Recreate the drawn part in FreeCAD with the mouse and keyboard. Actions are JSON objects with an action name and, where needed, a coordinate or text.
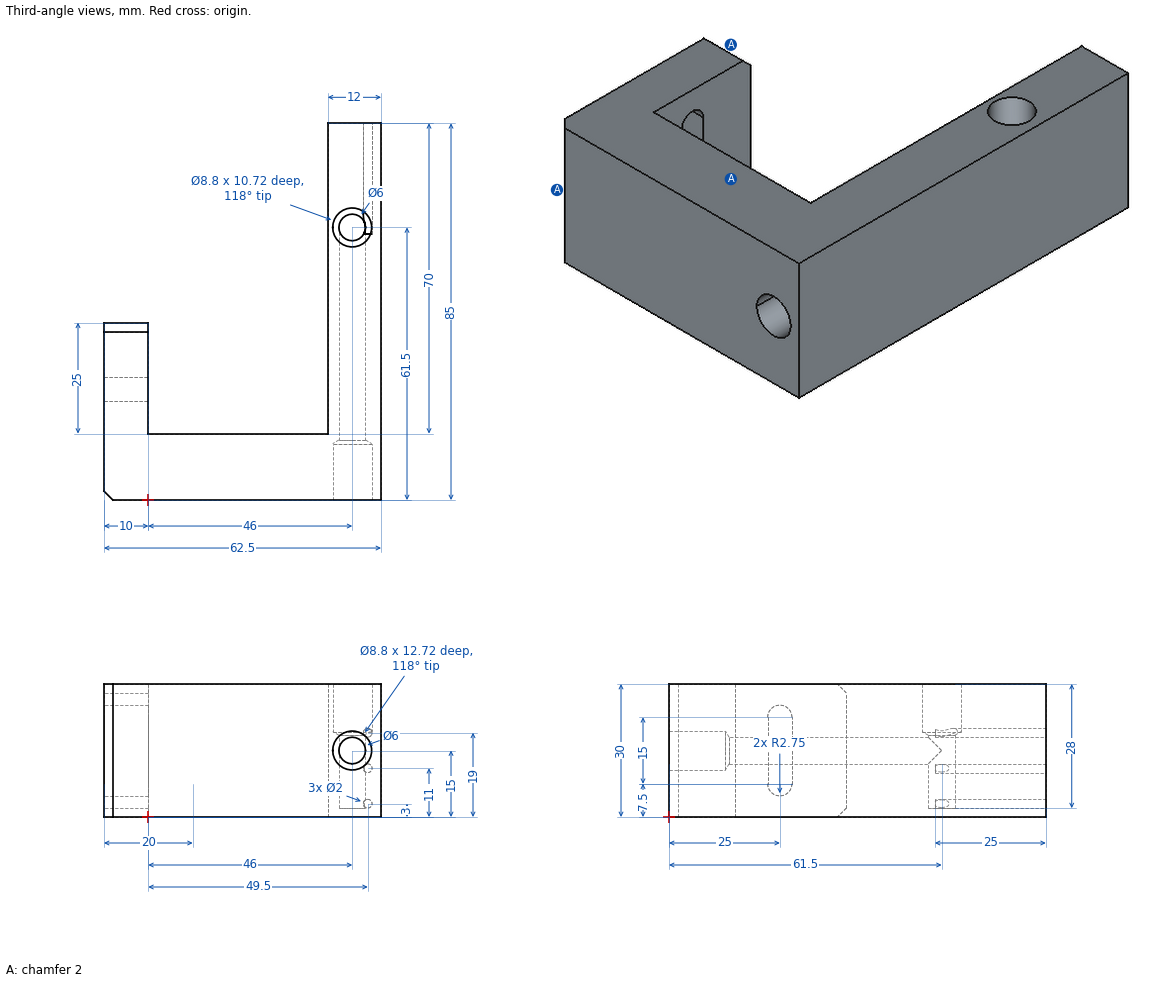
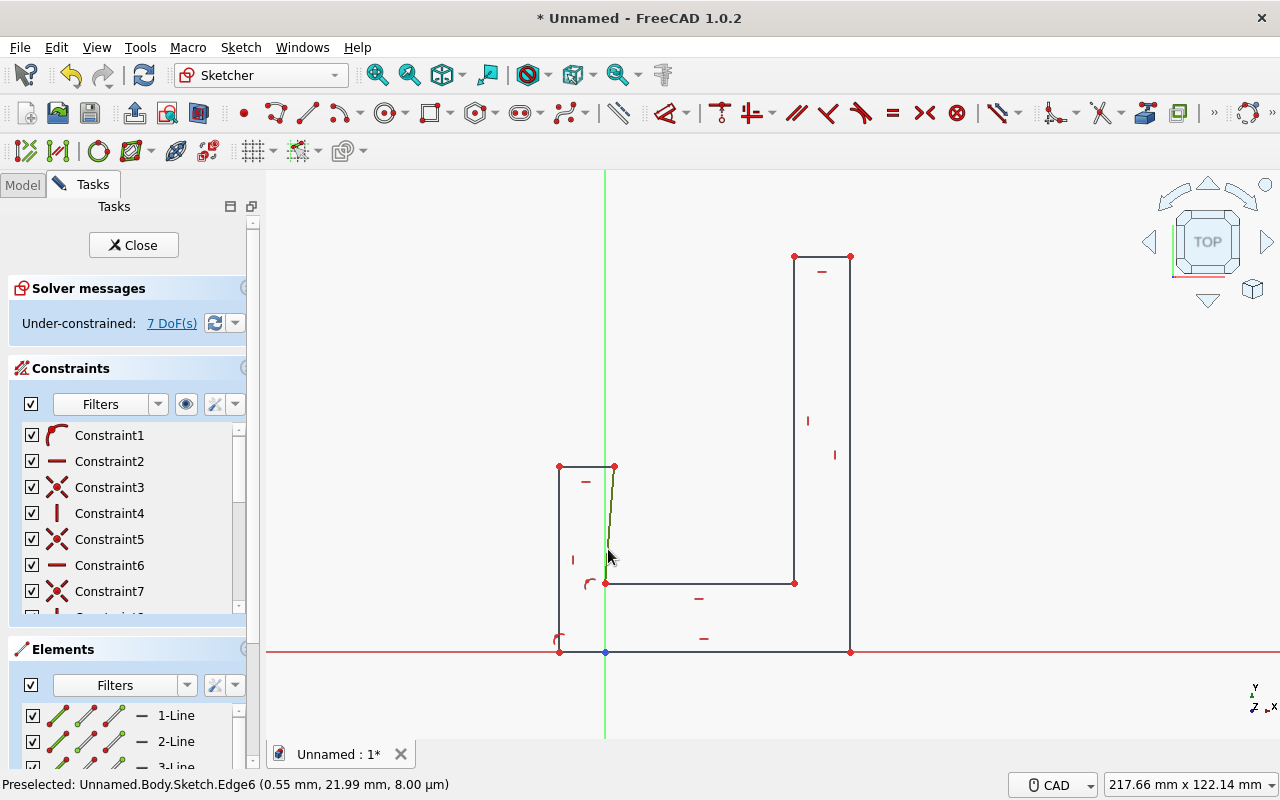
{"action": "left_click", "coordinate": [774, 114]}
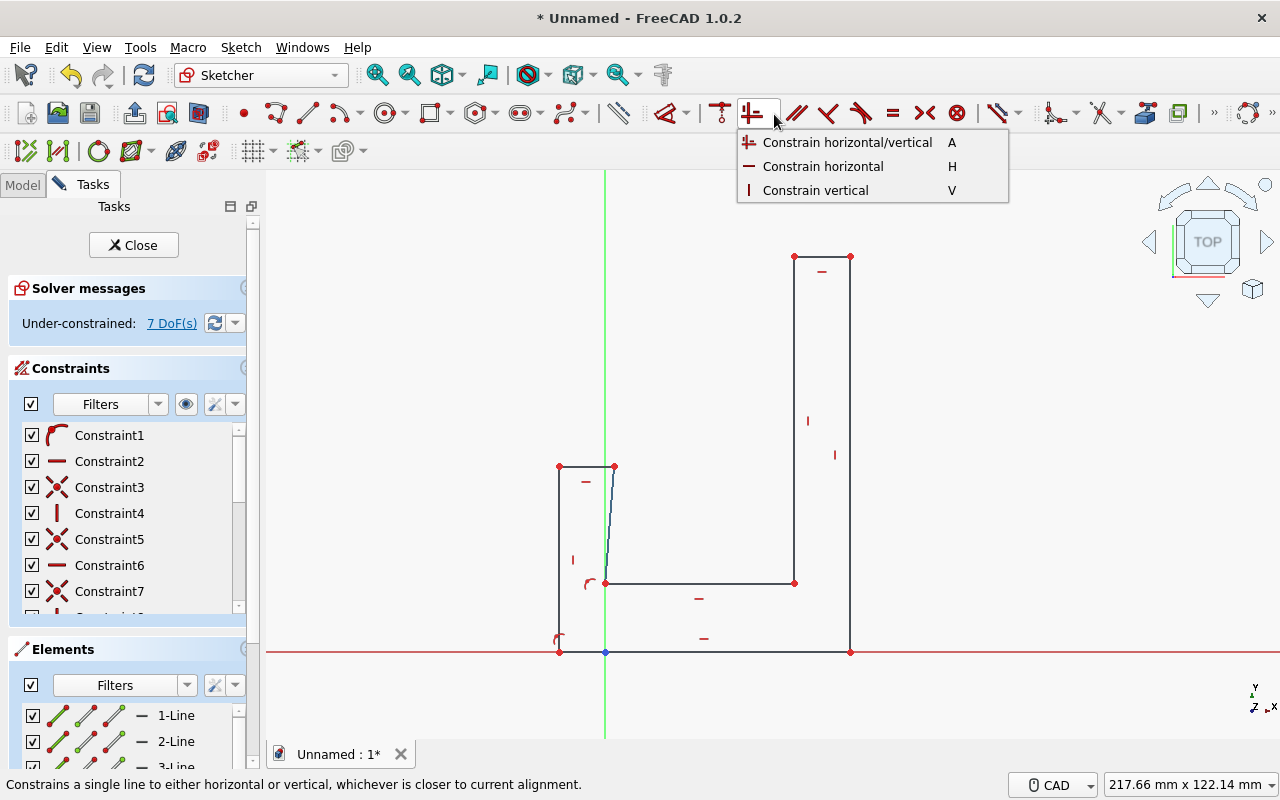
{"action": "left_click", "coordinate": [873, 190]}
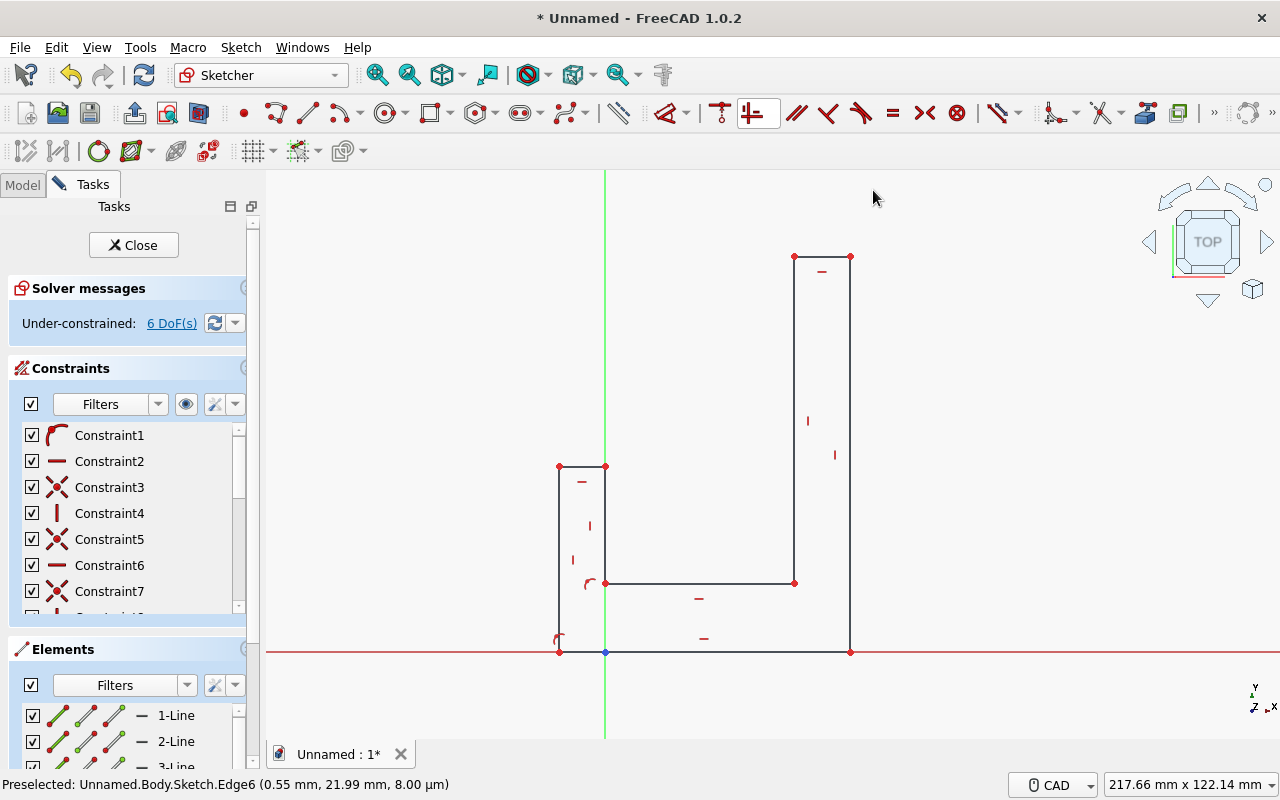
{"action": "left_click", "coordinate": [666, 114]}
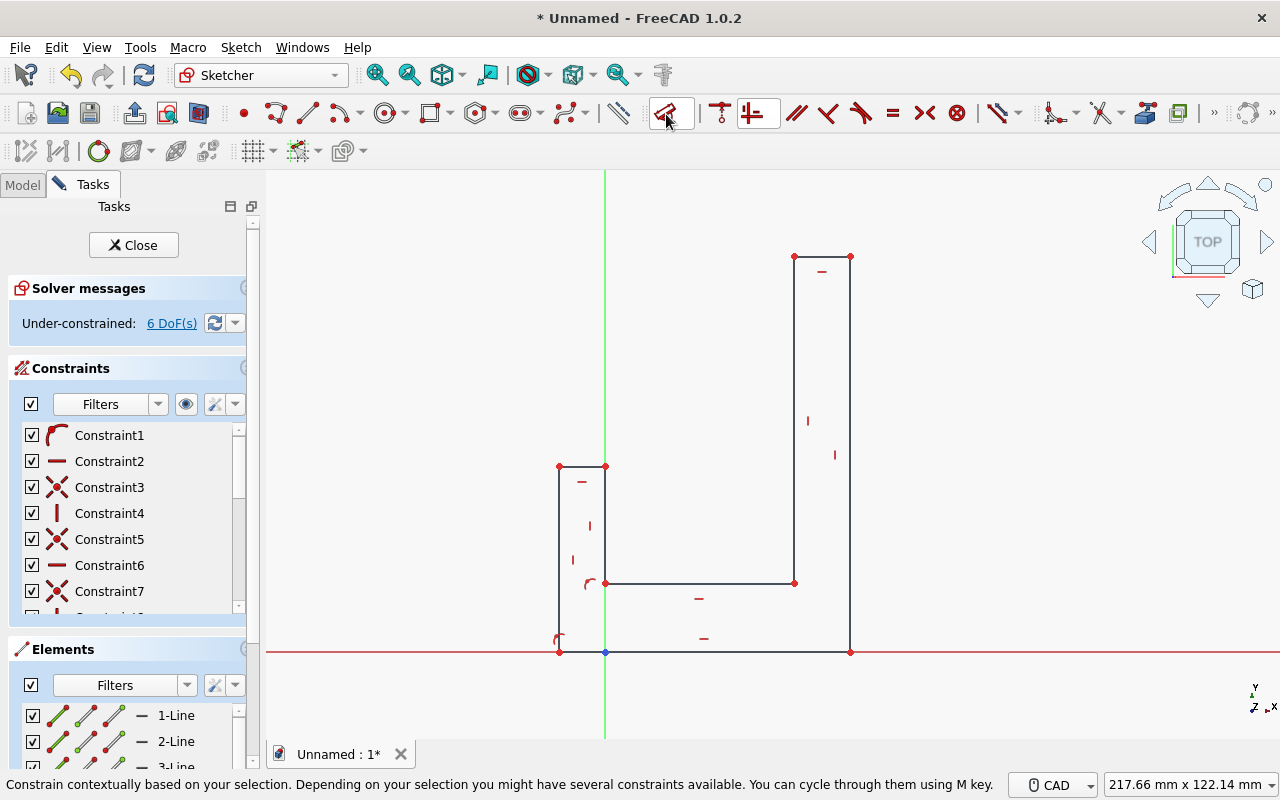
{"action": "left_click", "coordinate": [850, 534]}
{"action": "left_click", "coordinate": [884, 455]}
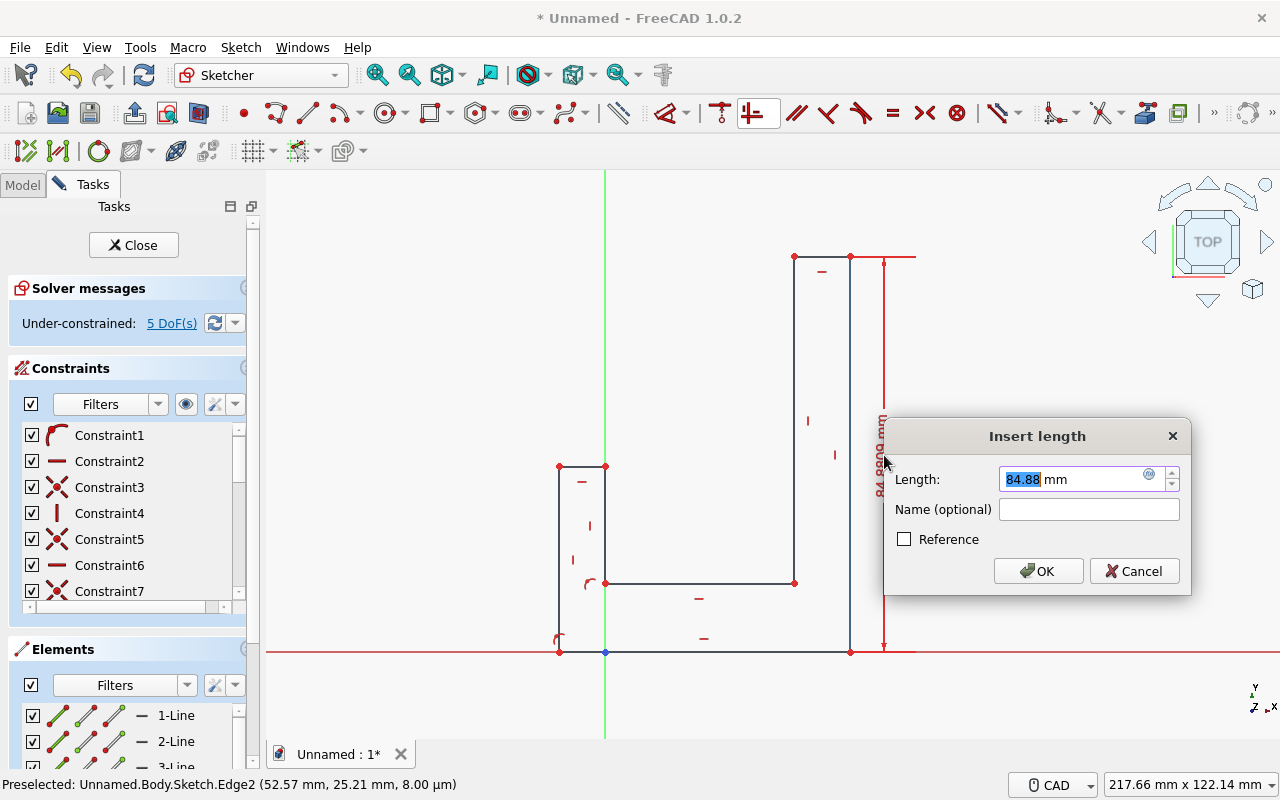
{"action": "type", "text": "85"}
{"action": "key", "text": "Return"}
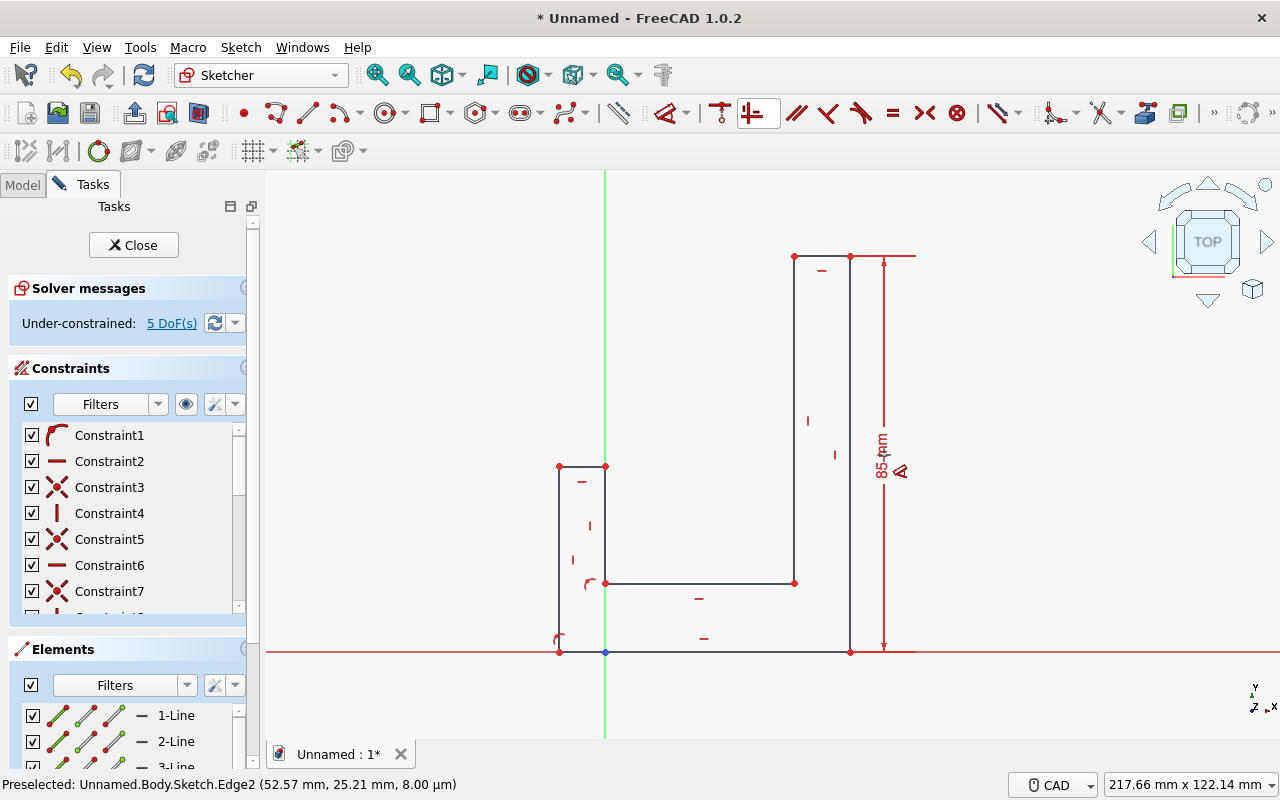
{"action": "left_click", "coordinate": [833, 256]}
{"action": "left_click", "coordinate": [822, 222]}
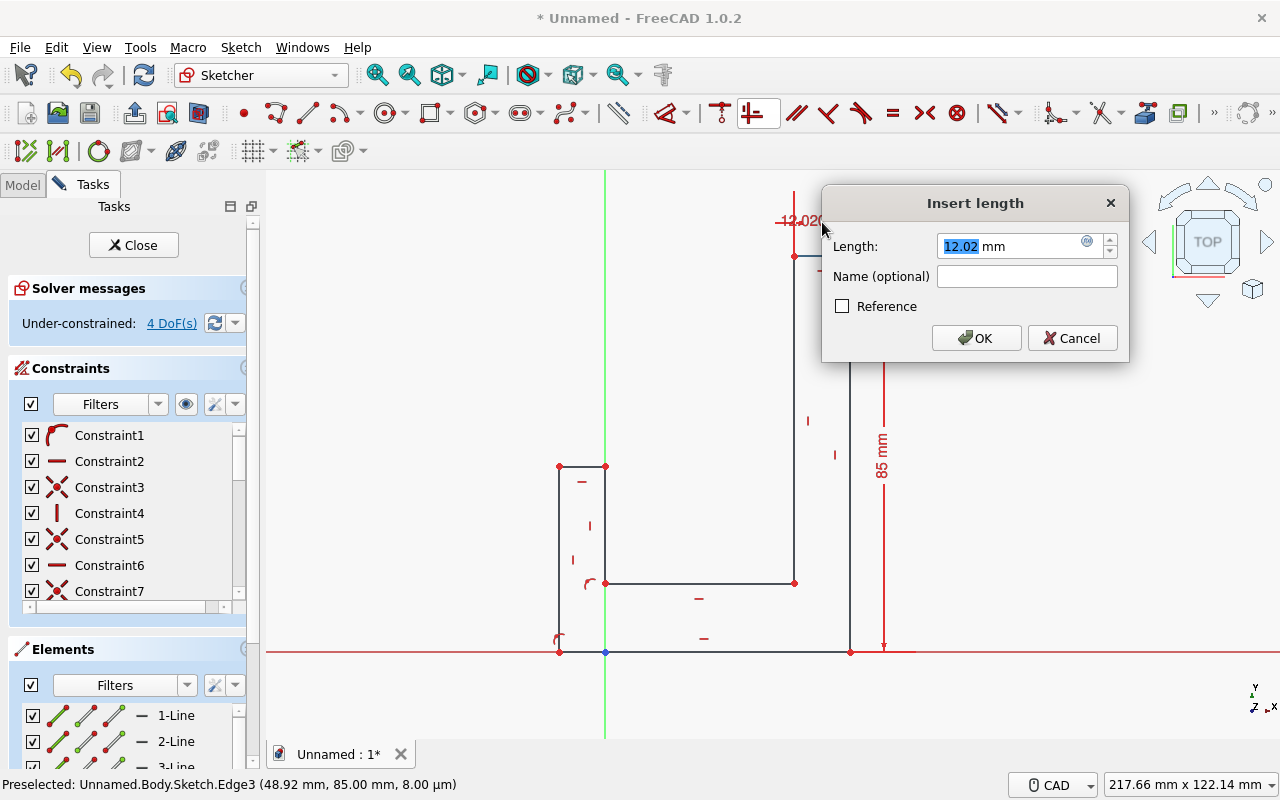
{"action": "type", "text": "12"}
{"action": "key", "text": "Return"}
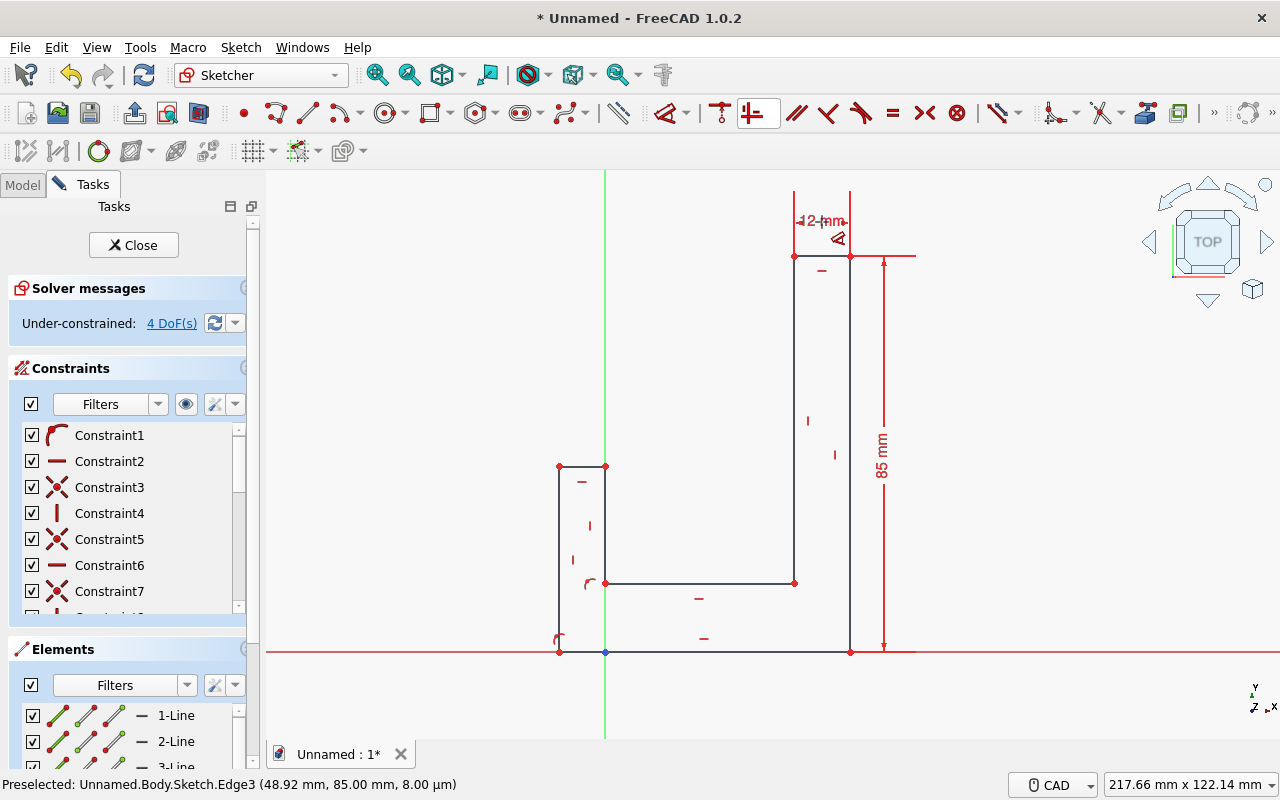
{"action": "left_click", "coordinate": [794, 355]}
{"action": "left_click", "coordinate": [828, 420]}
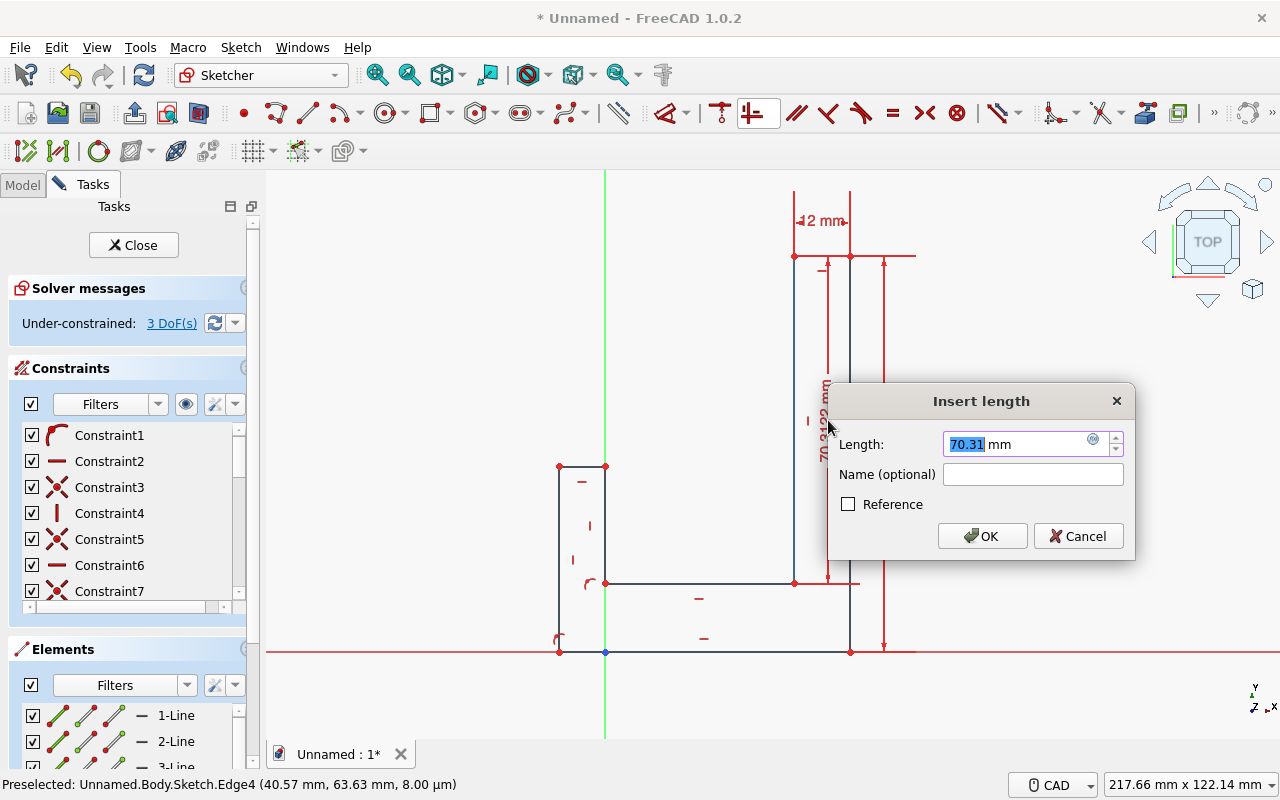
{"action": "type", "text": "70"}
{"action": "key", "text": "Return"}